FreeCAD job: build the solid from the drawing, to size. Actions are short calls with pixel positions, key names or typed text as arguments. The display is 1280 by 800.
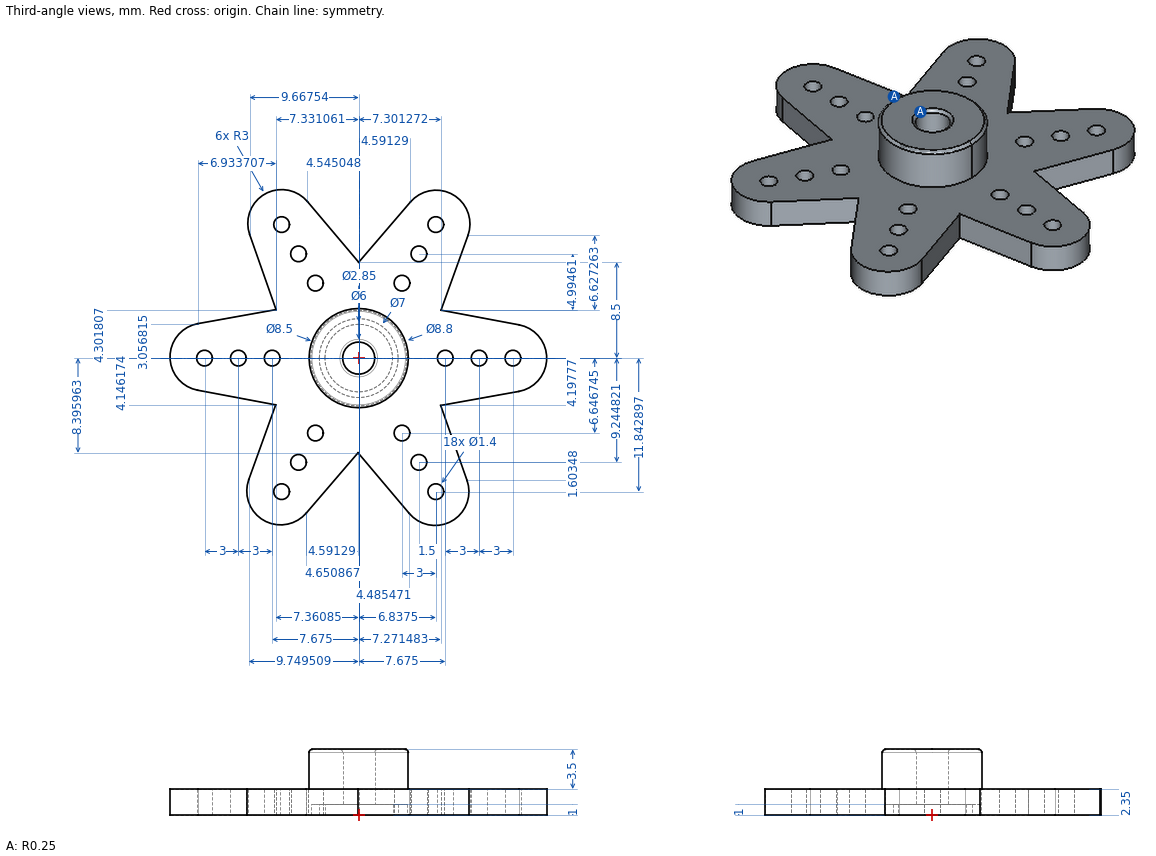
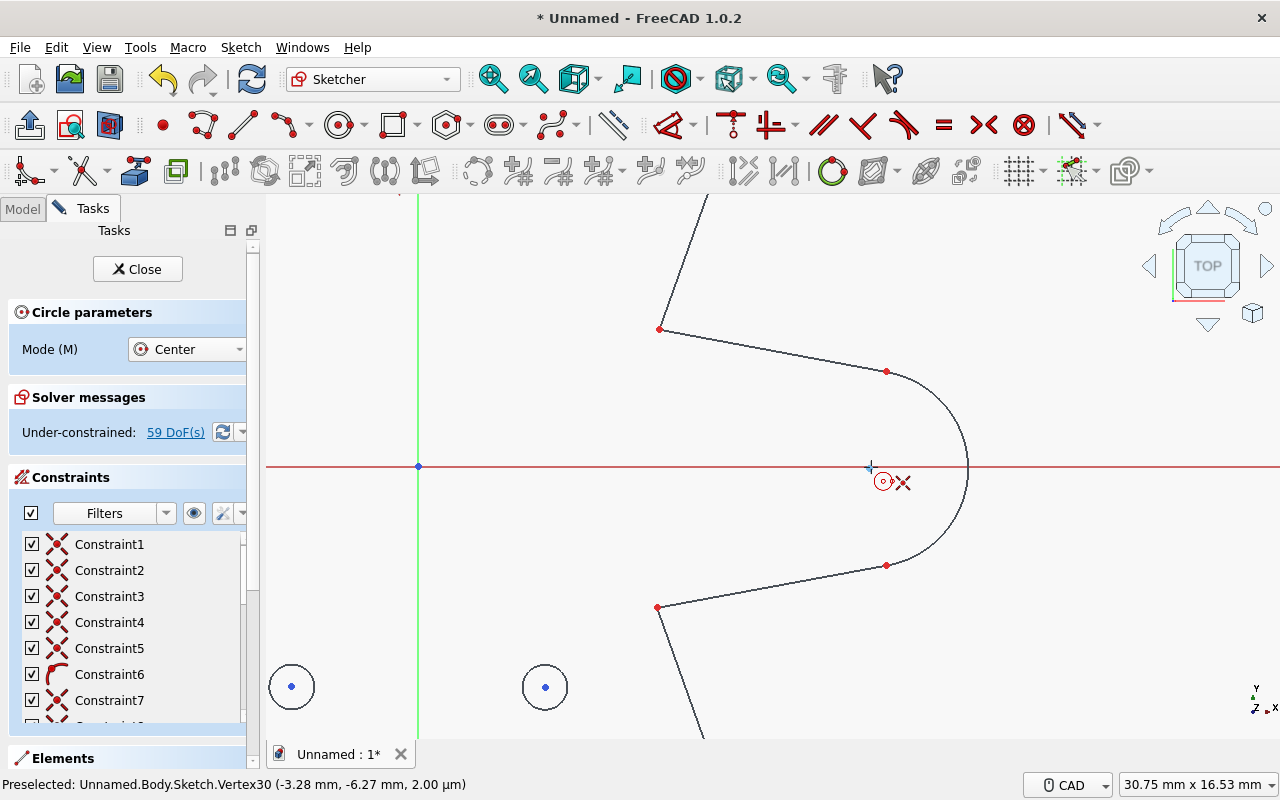
click(869, 467)
click(885, 451)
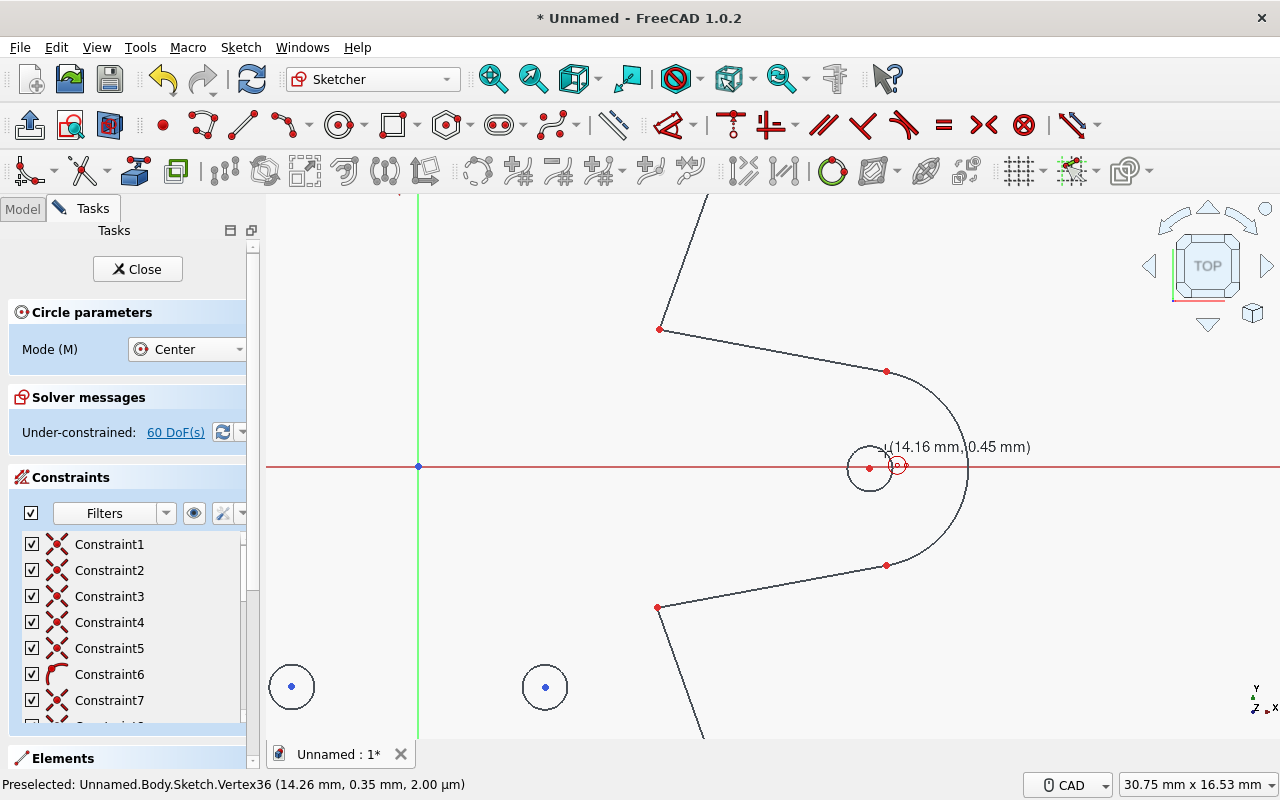
click(770, 467)
click(786, 451)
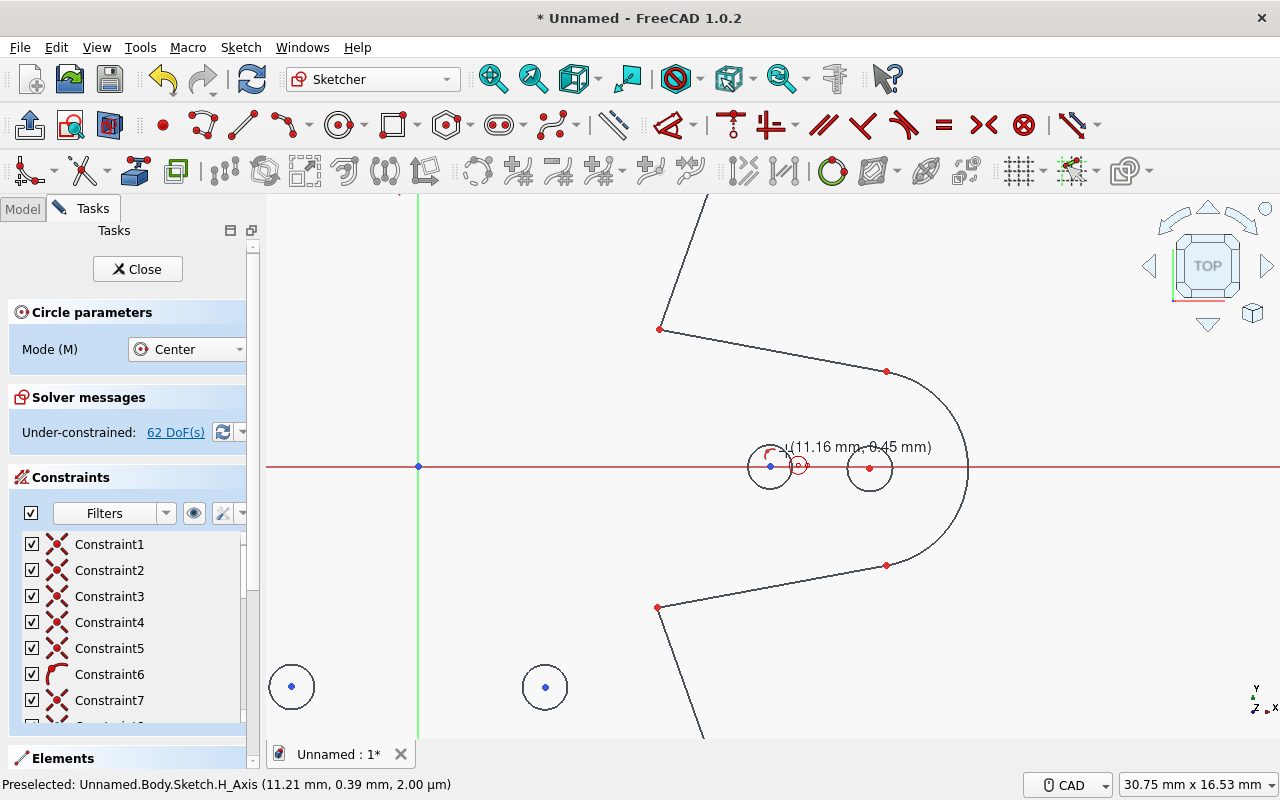
click(671, 467)
click(688, 451)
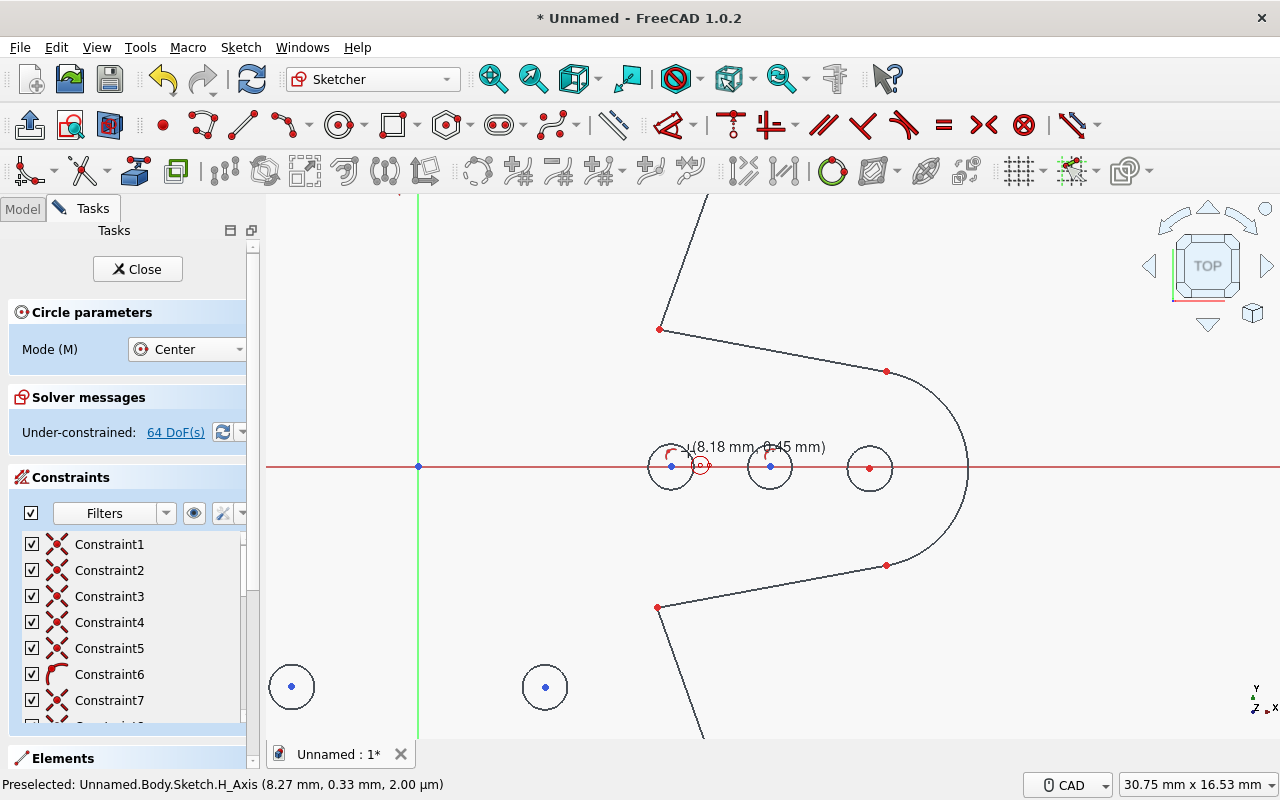
click(545, 248)
click(561, 232)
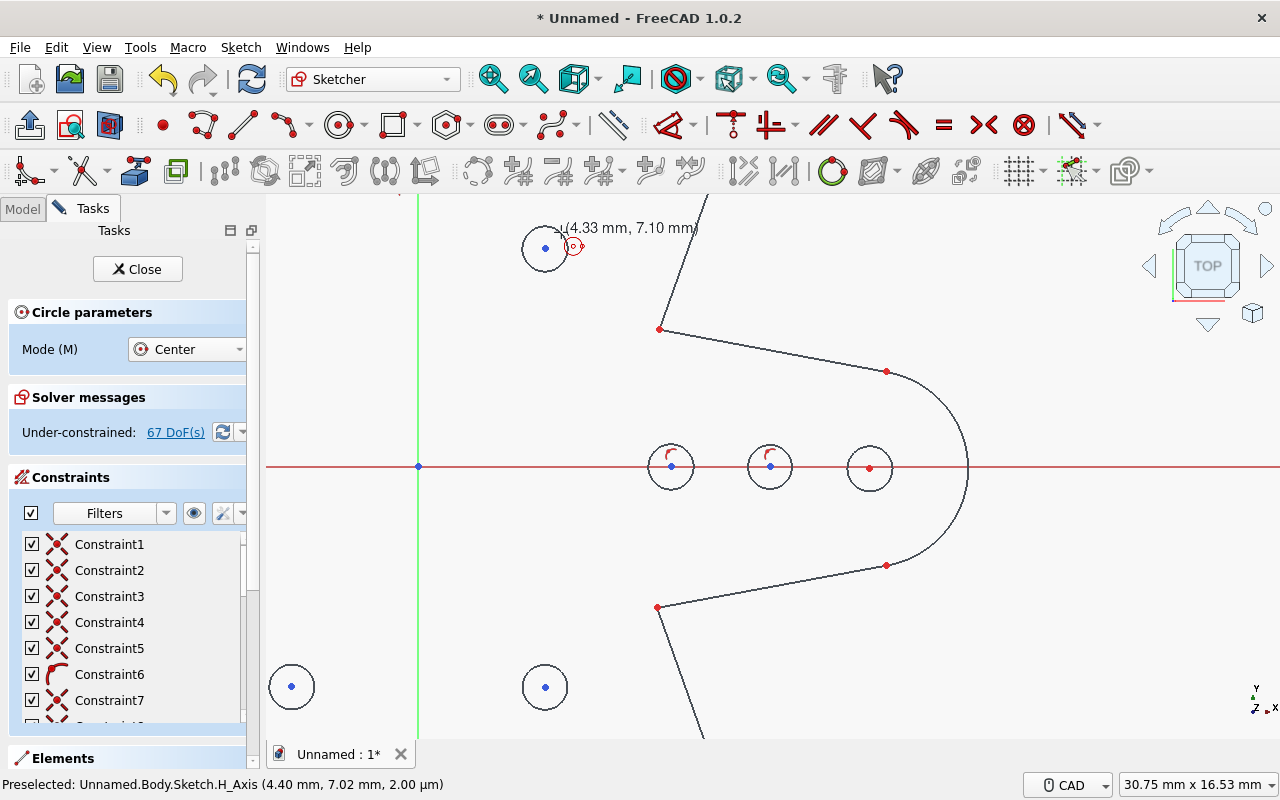
scroll(872, 467, down, 5)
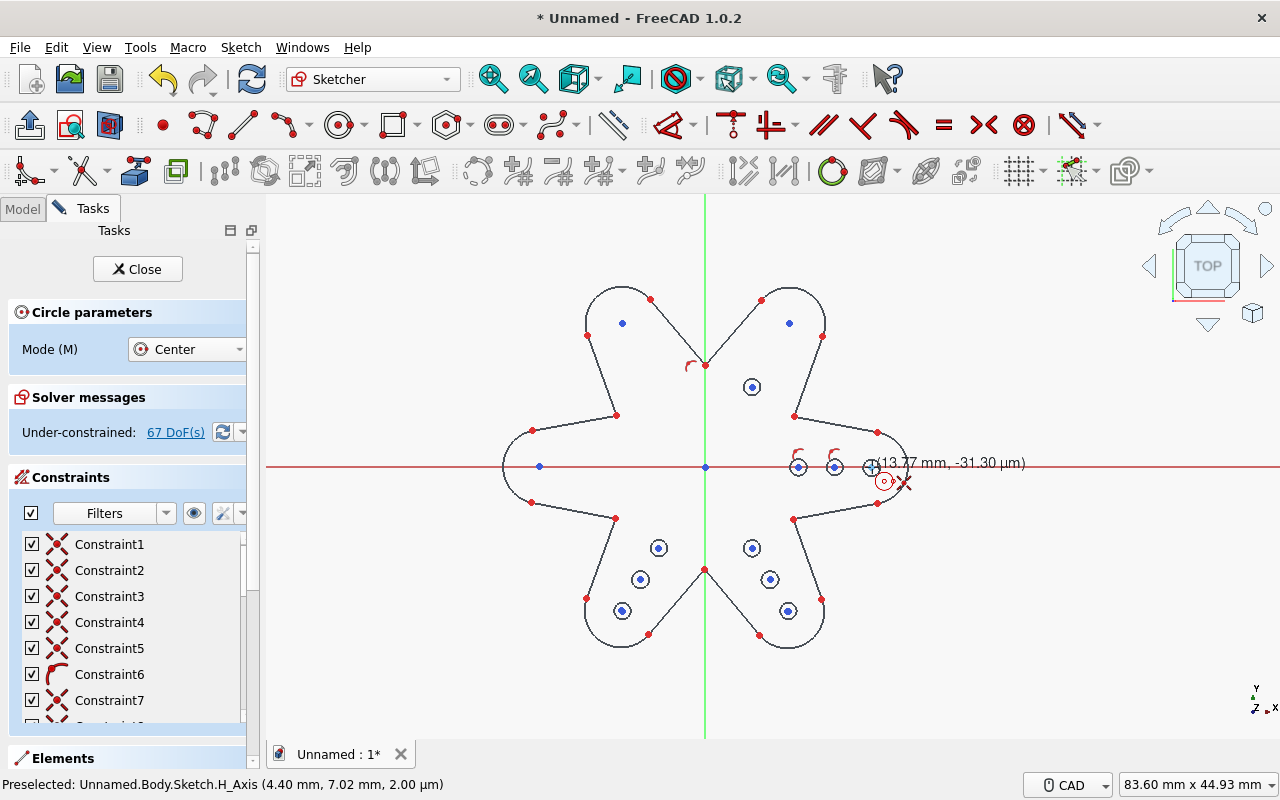
scroll(770, 355, up, 5)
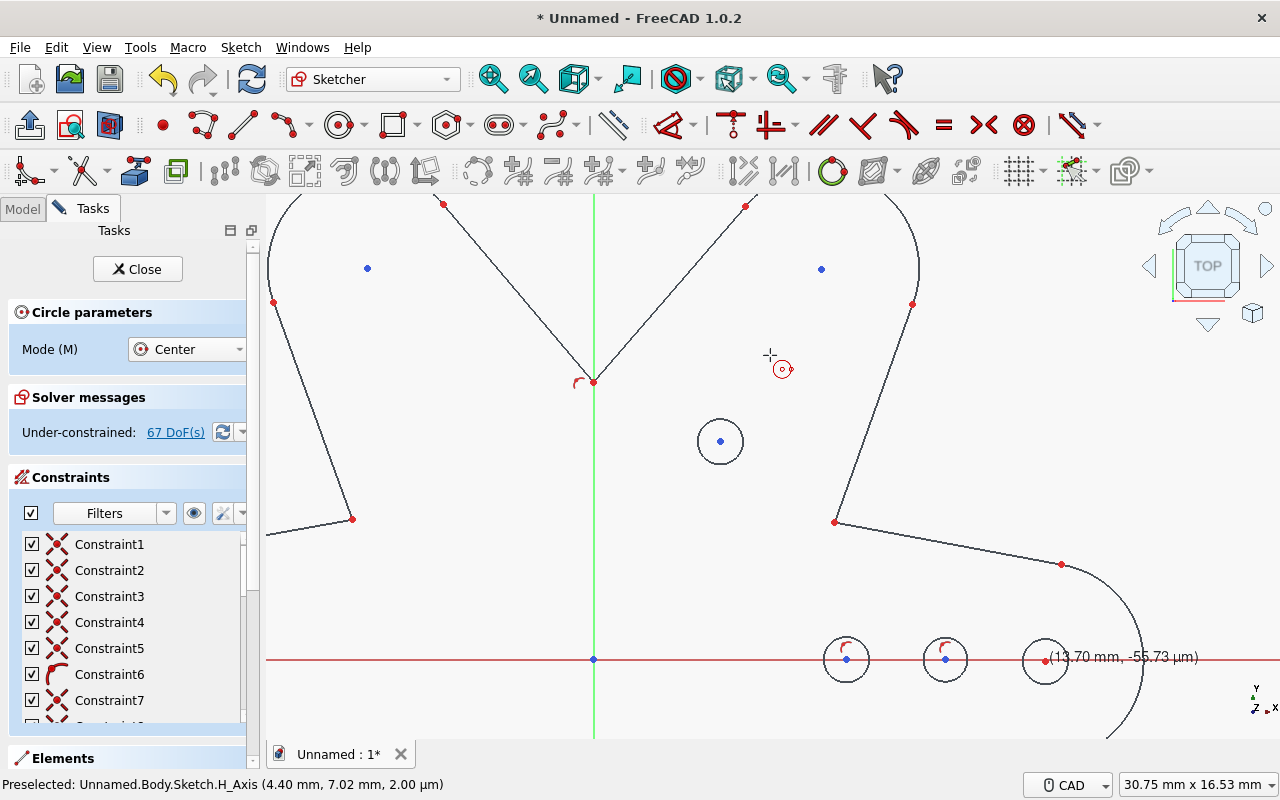
click(770, 355)
click(786, 339)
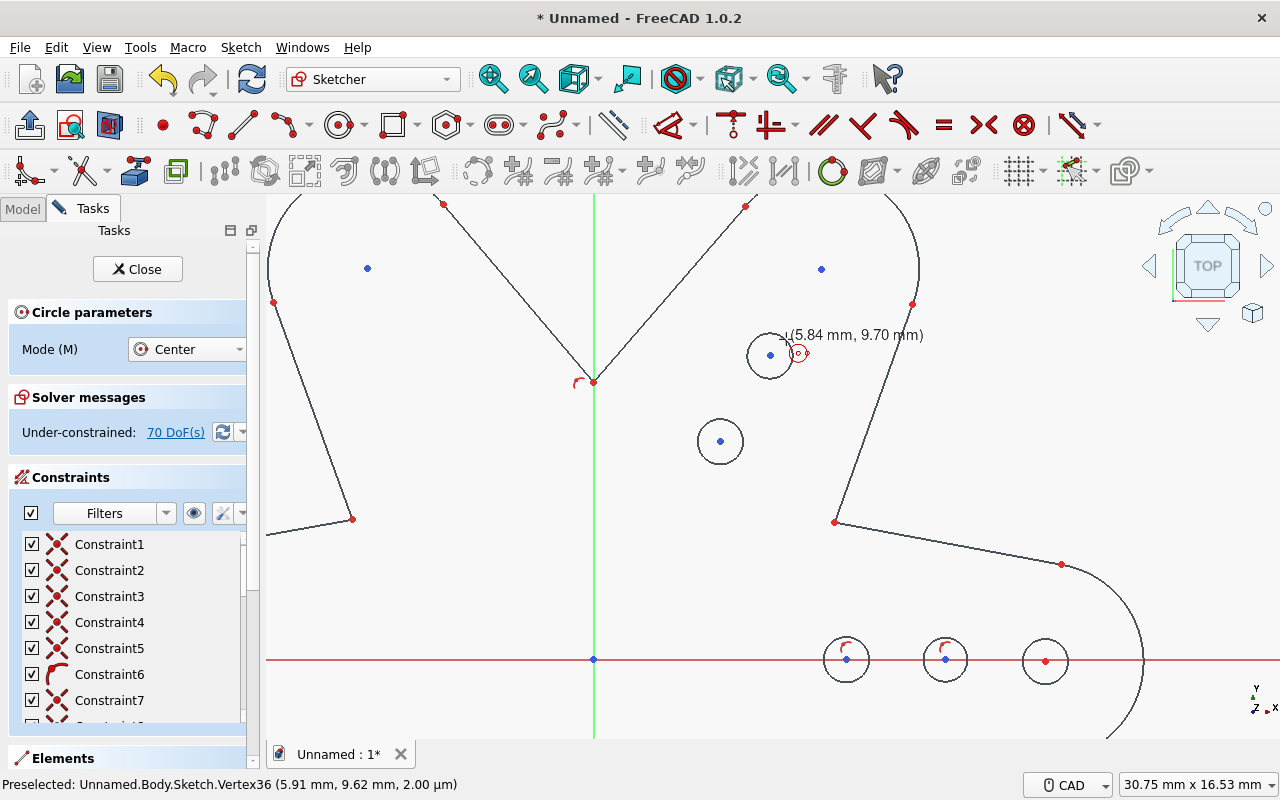
scroll(819, 269, up, 11)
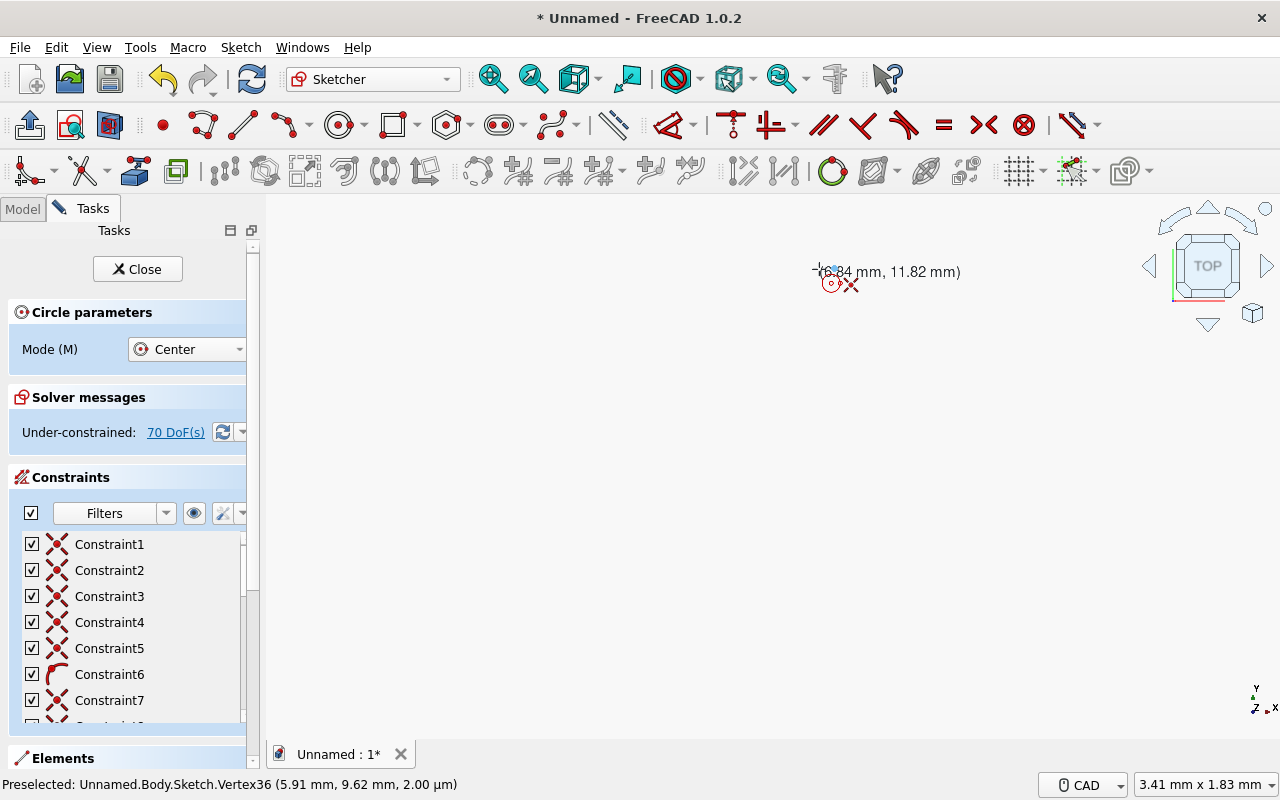
click(815, 271)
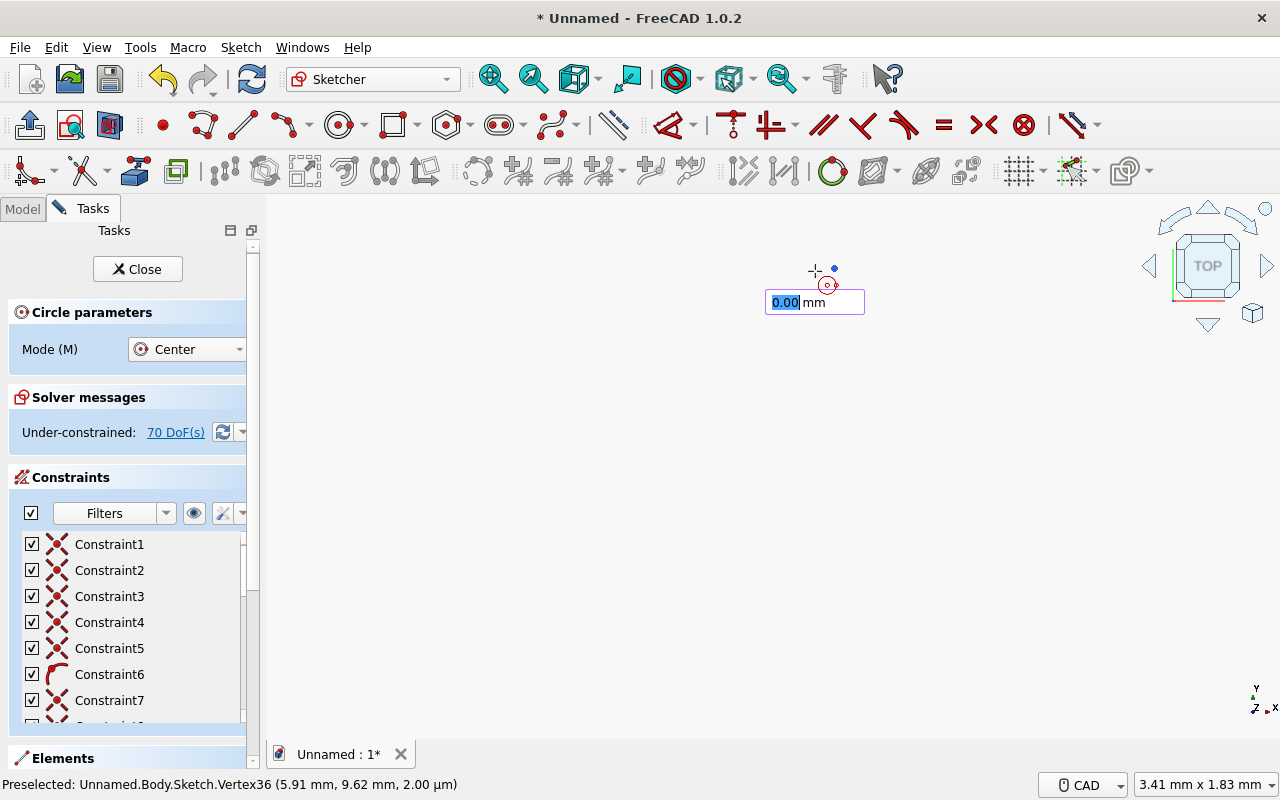
scroll(806, 293, down, 15)